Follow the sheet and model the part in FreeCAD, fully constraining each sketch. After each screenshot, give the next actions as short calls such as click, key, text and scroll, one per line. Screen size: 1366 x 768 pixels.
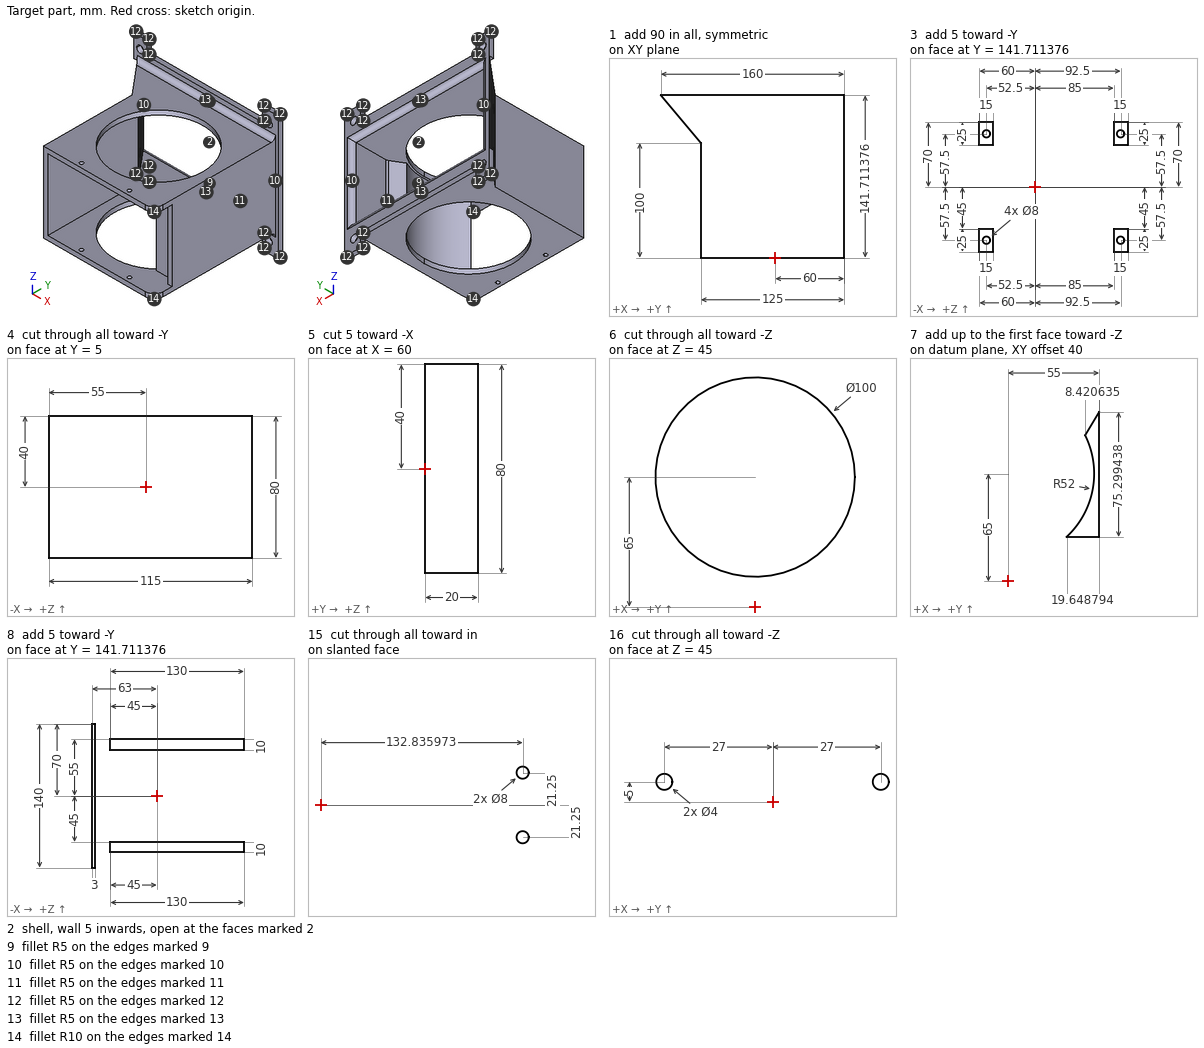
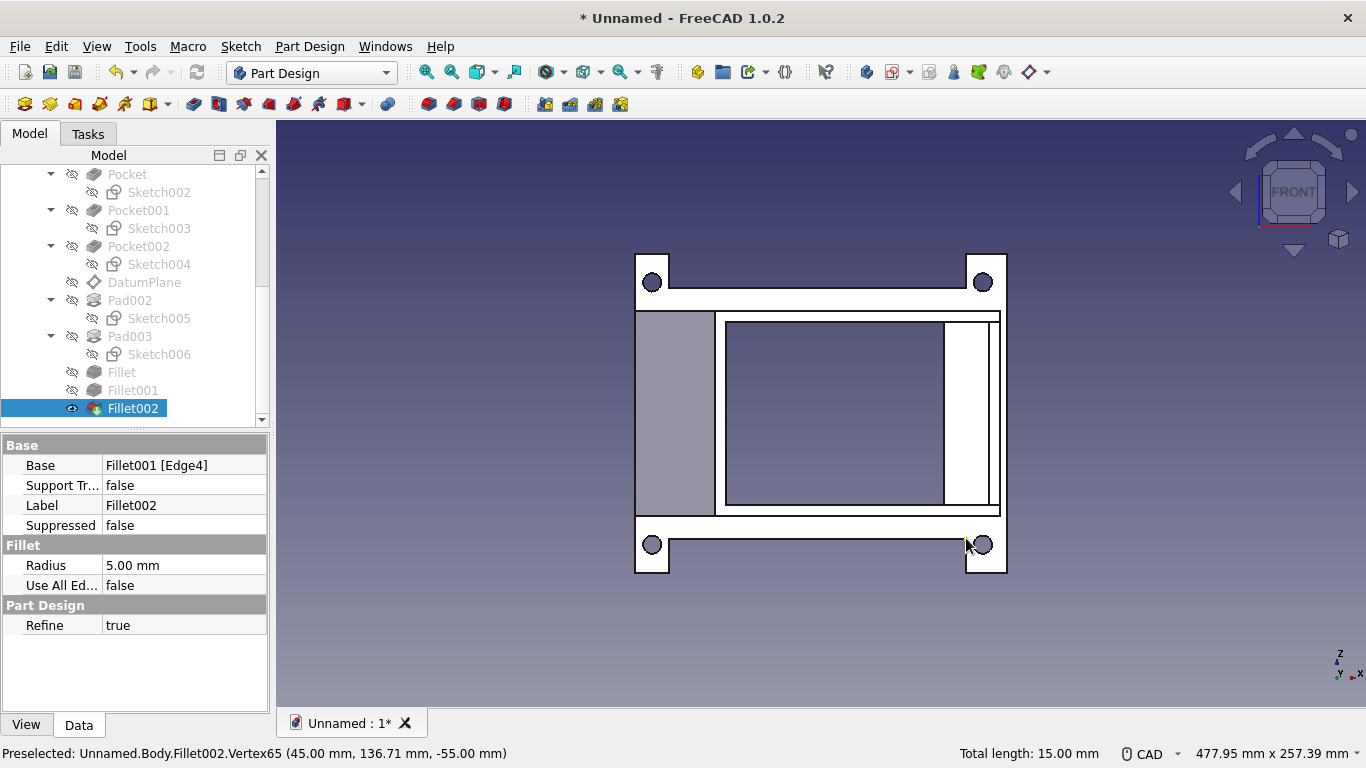
key(3)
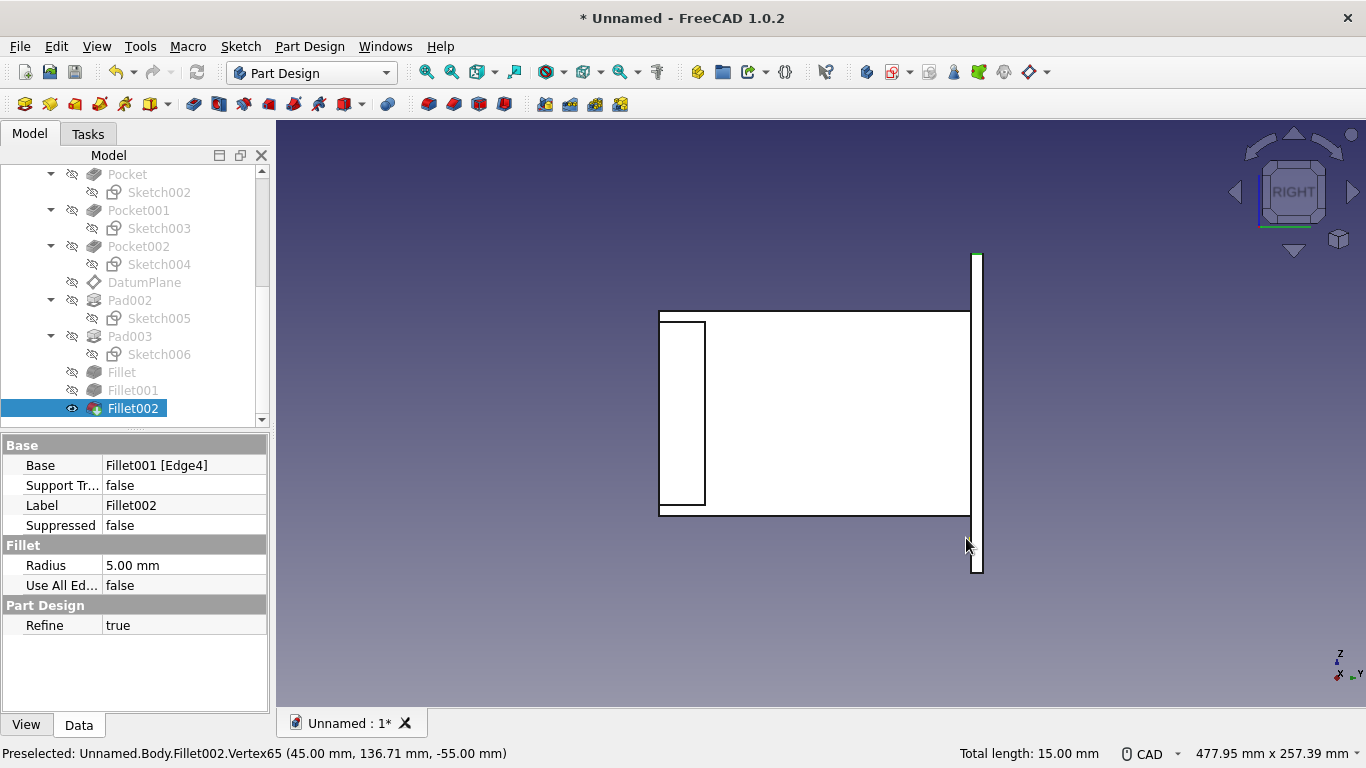
scroll(977, 538, up, 7)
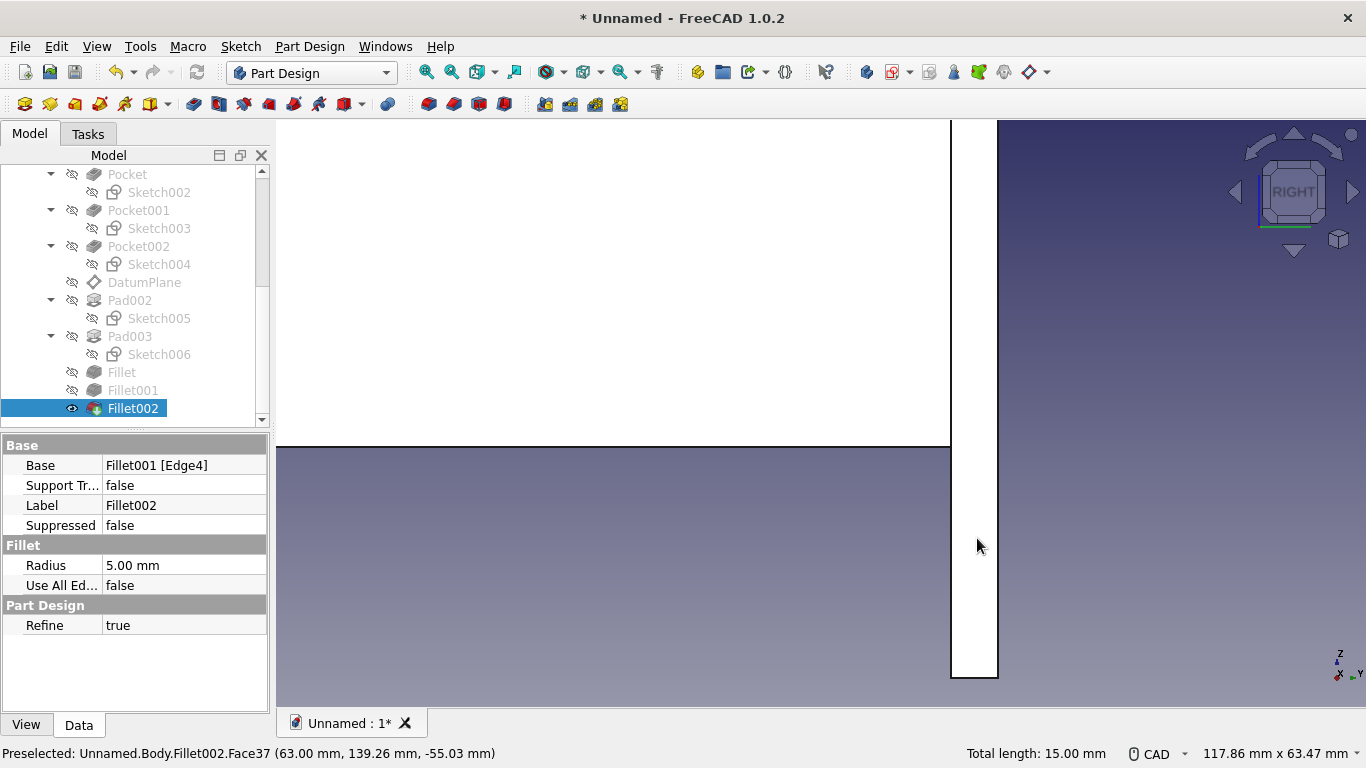
click(975, 677, ctrl)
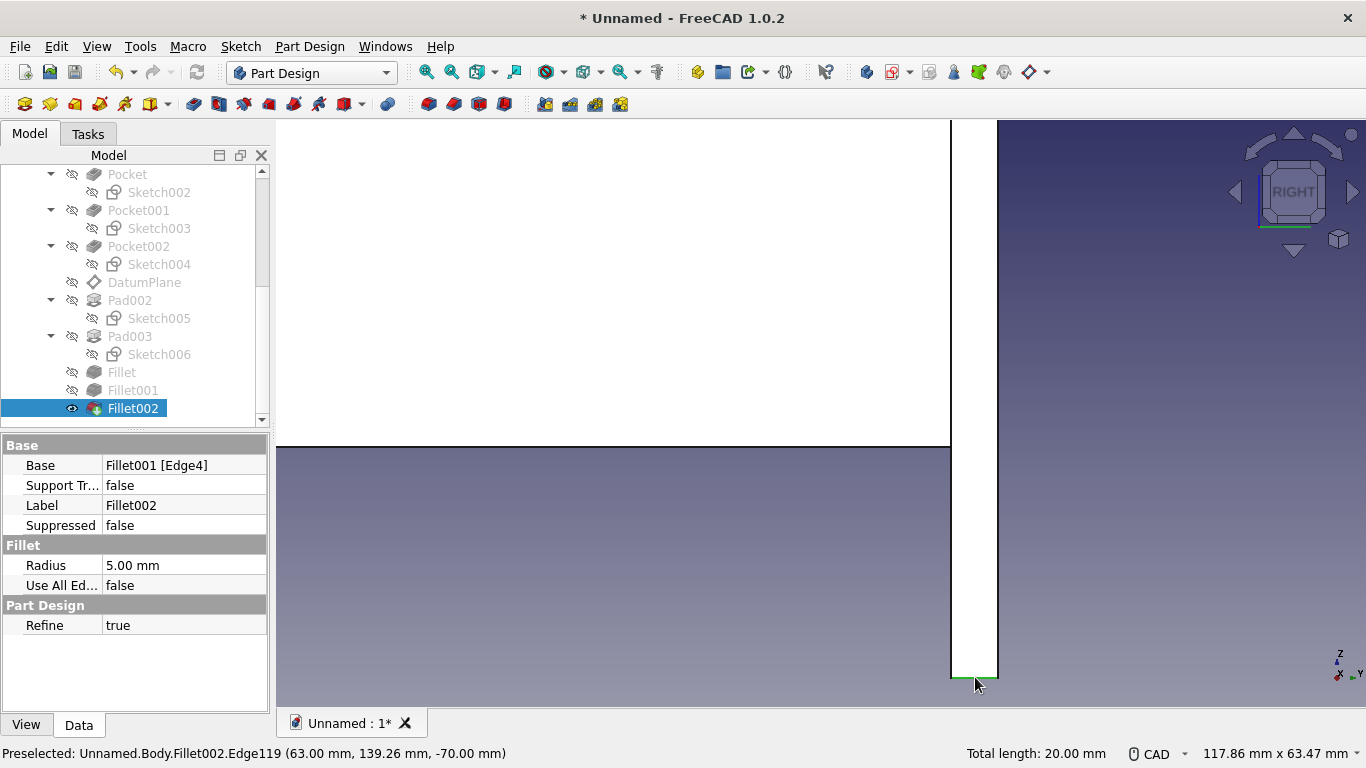
click(427, 72)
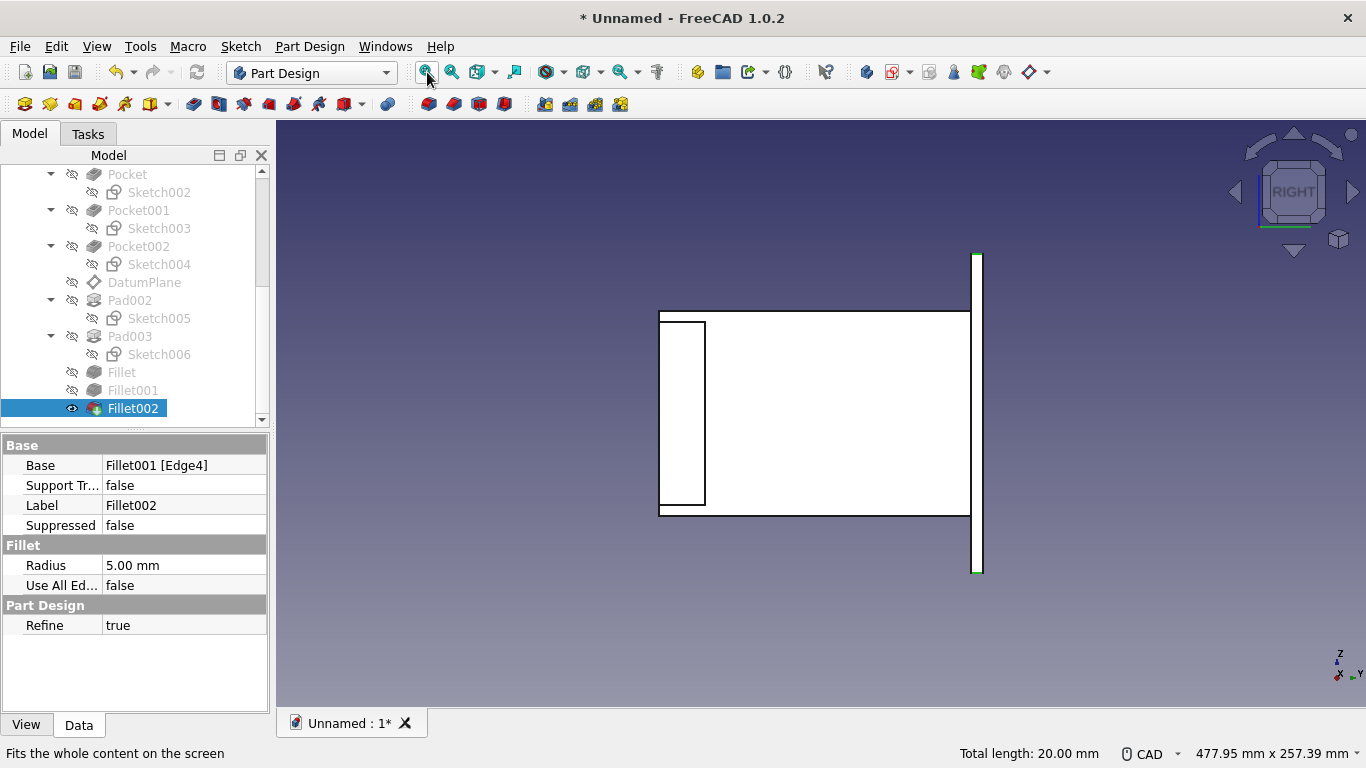
key(5)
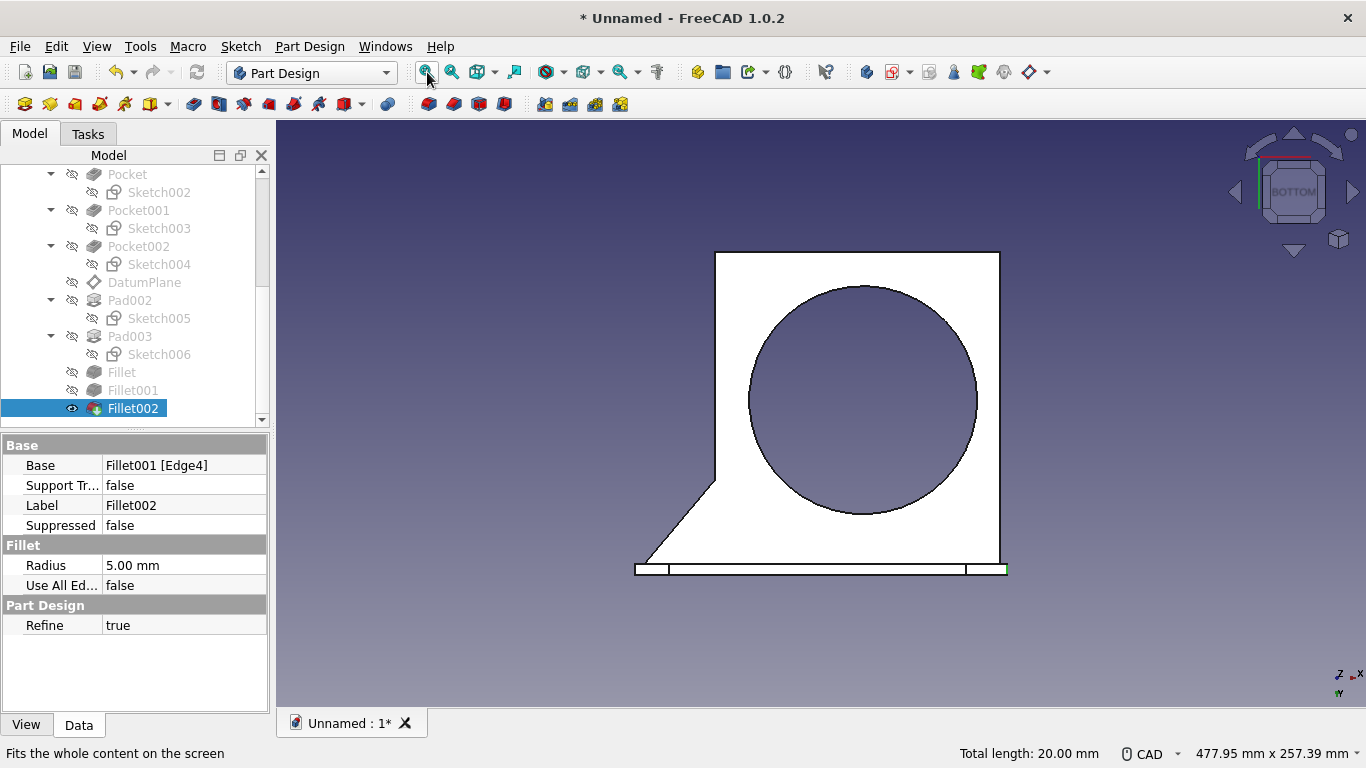
scroll(966, 568, up, 7)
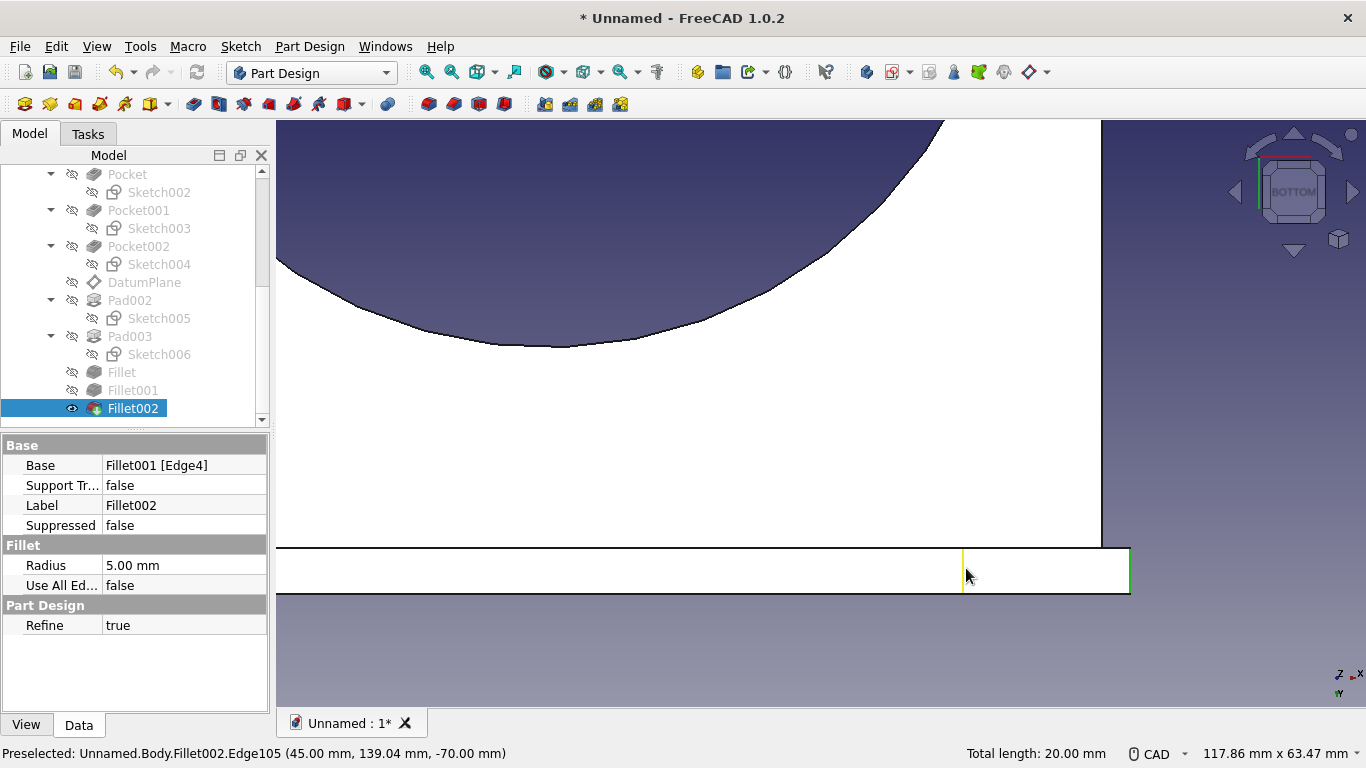
click(963, 570, ctrl)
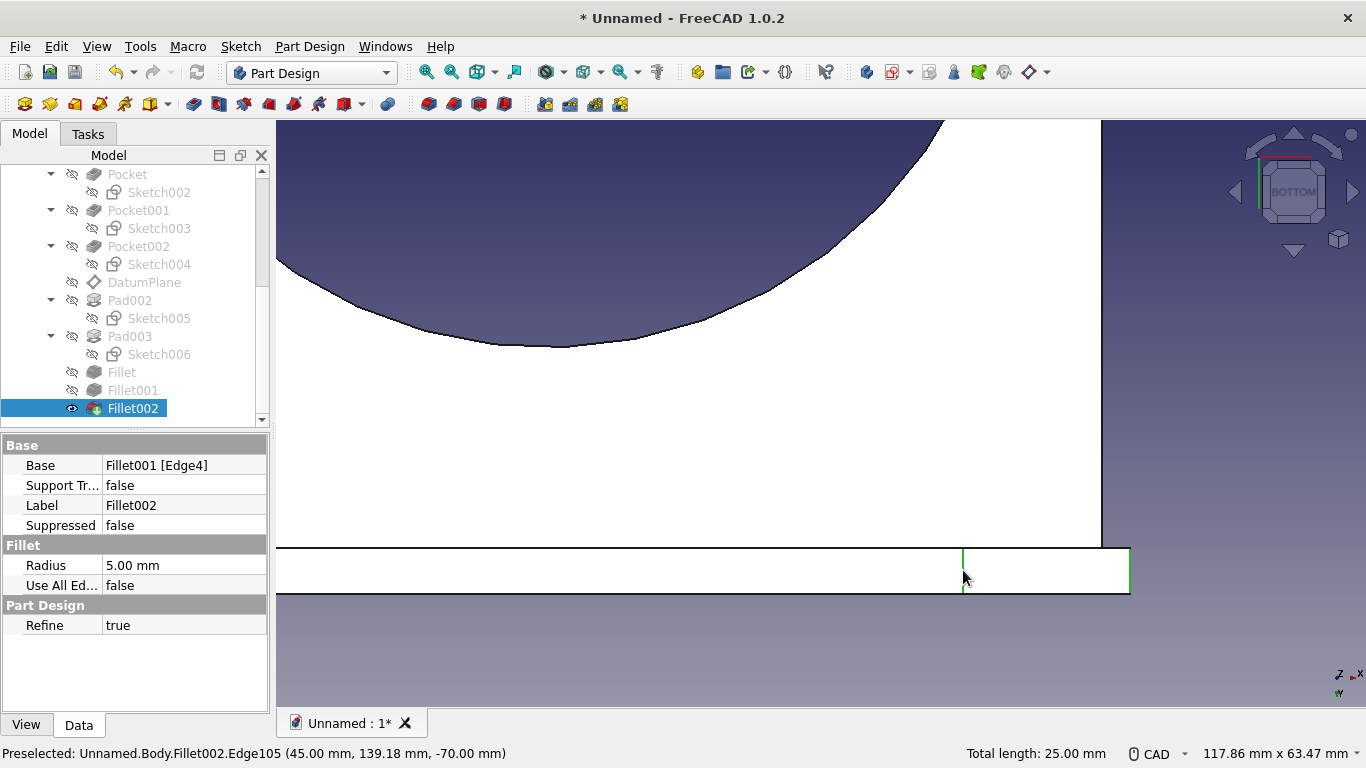
key(v)
key(f)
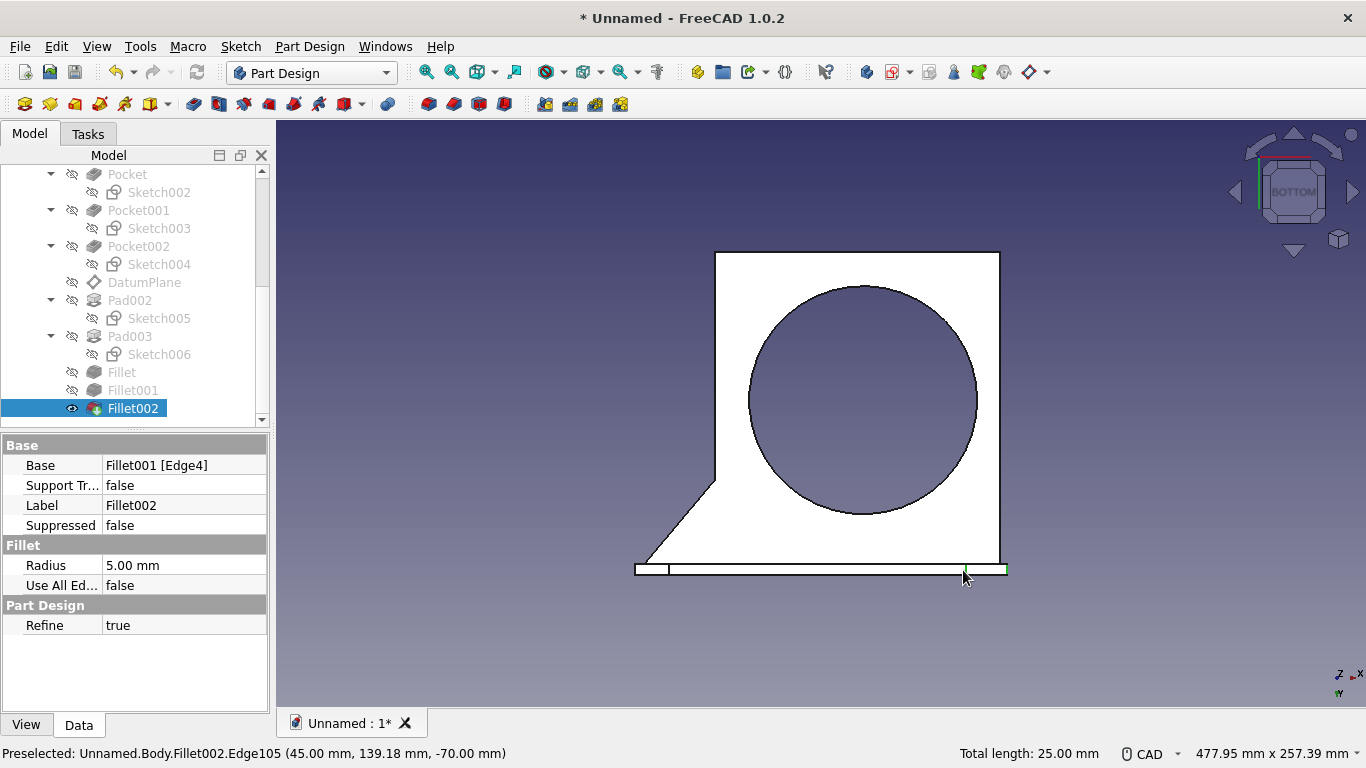
key(4)